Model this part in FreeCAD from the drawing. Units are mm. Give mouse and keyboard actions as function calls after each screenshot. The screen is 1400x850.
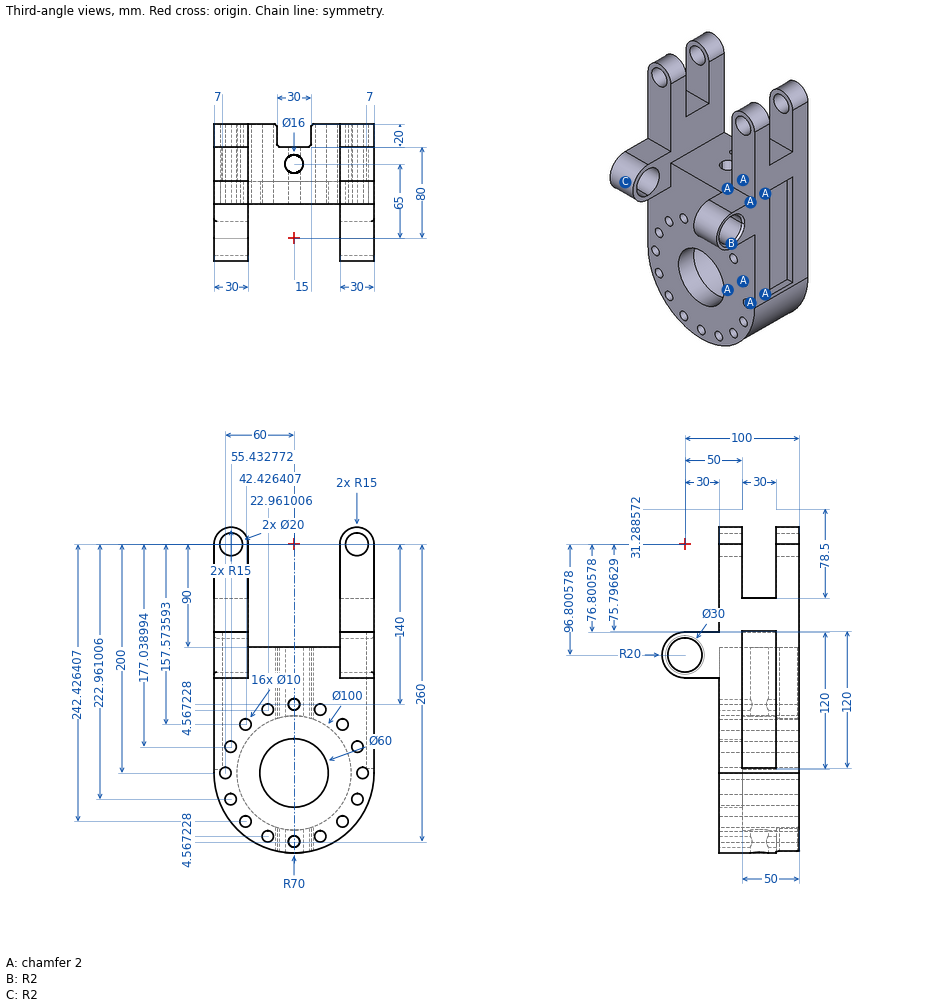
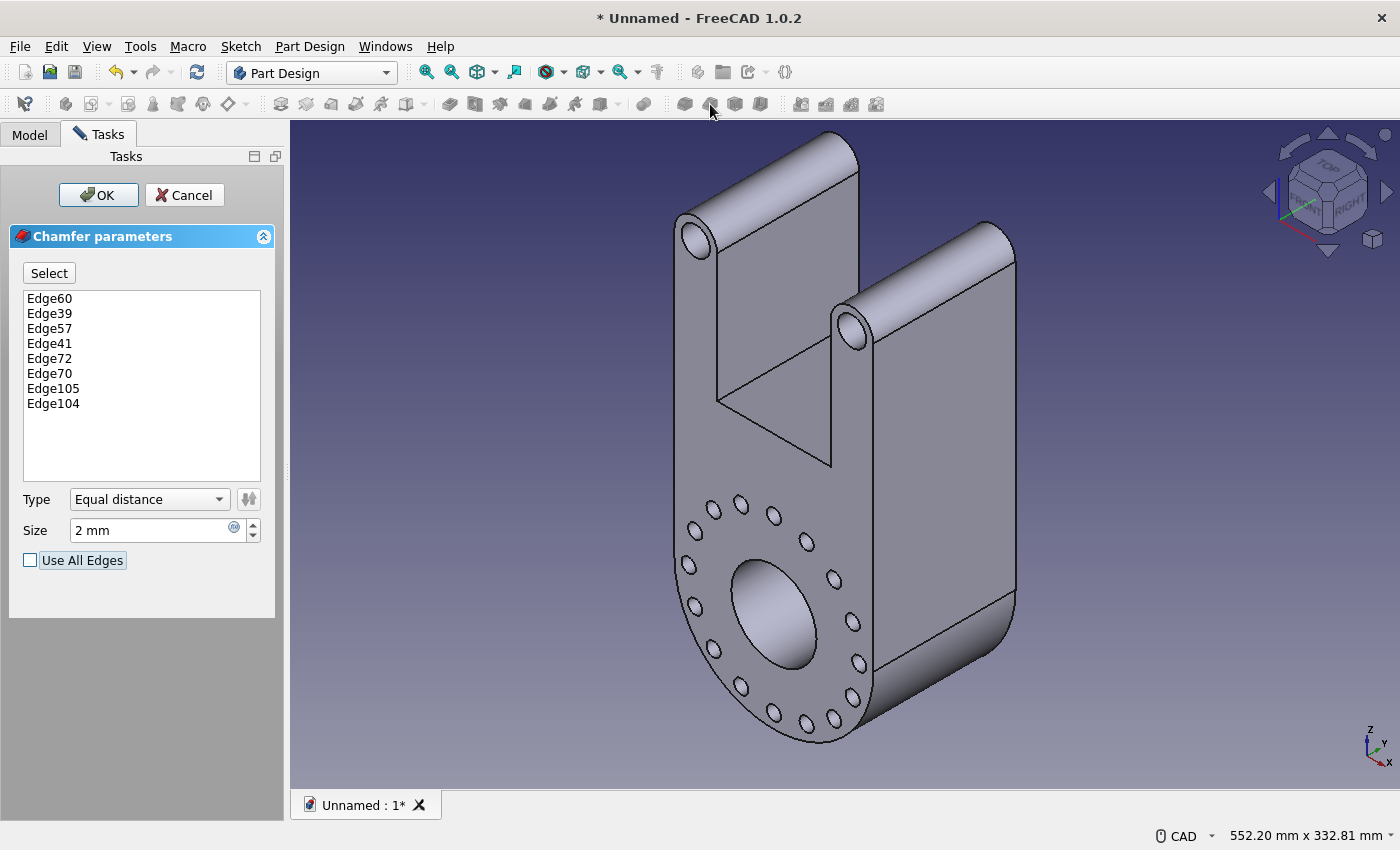
click(99, 195)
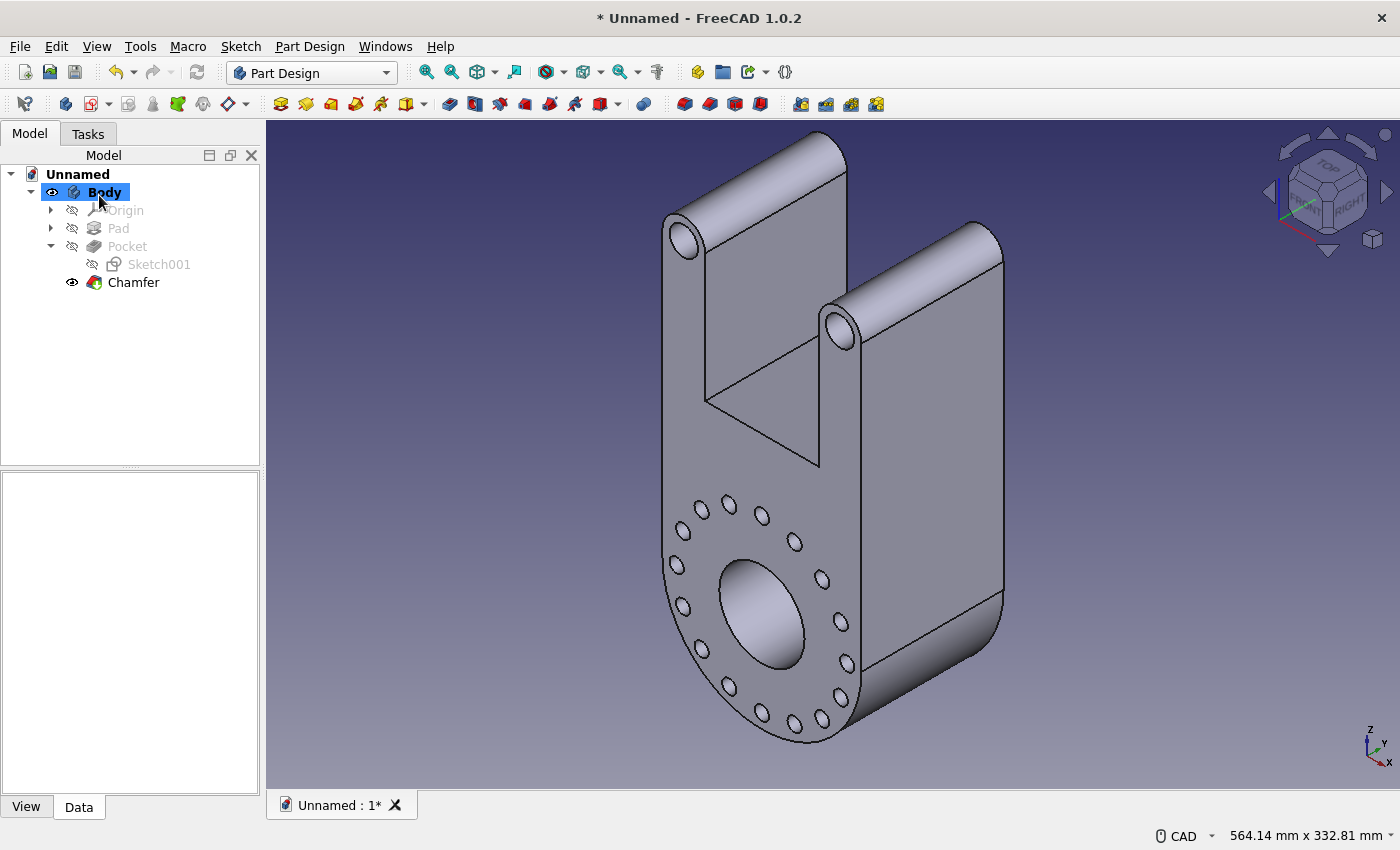
click(90, 104)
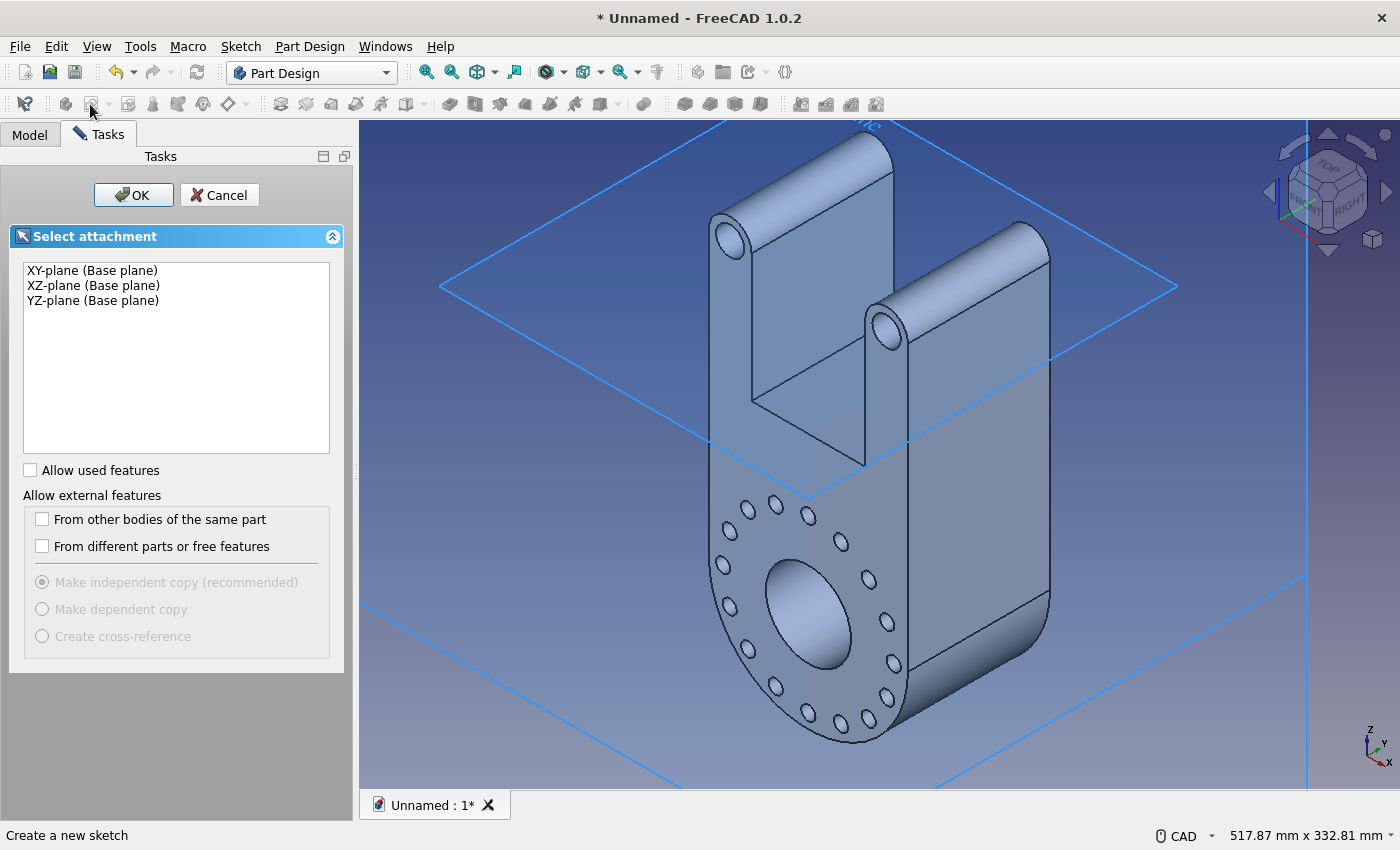
click(84, 286)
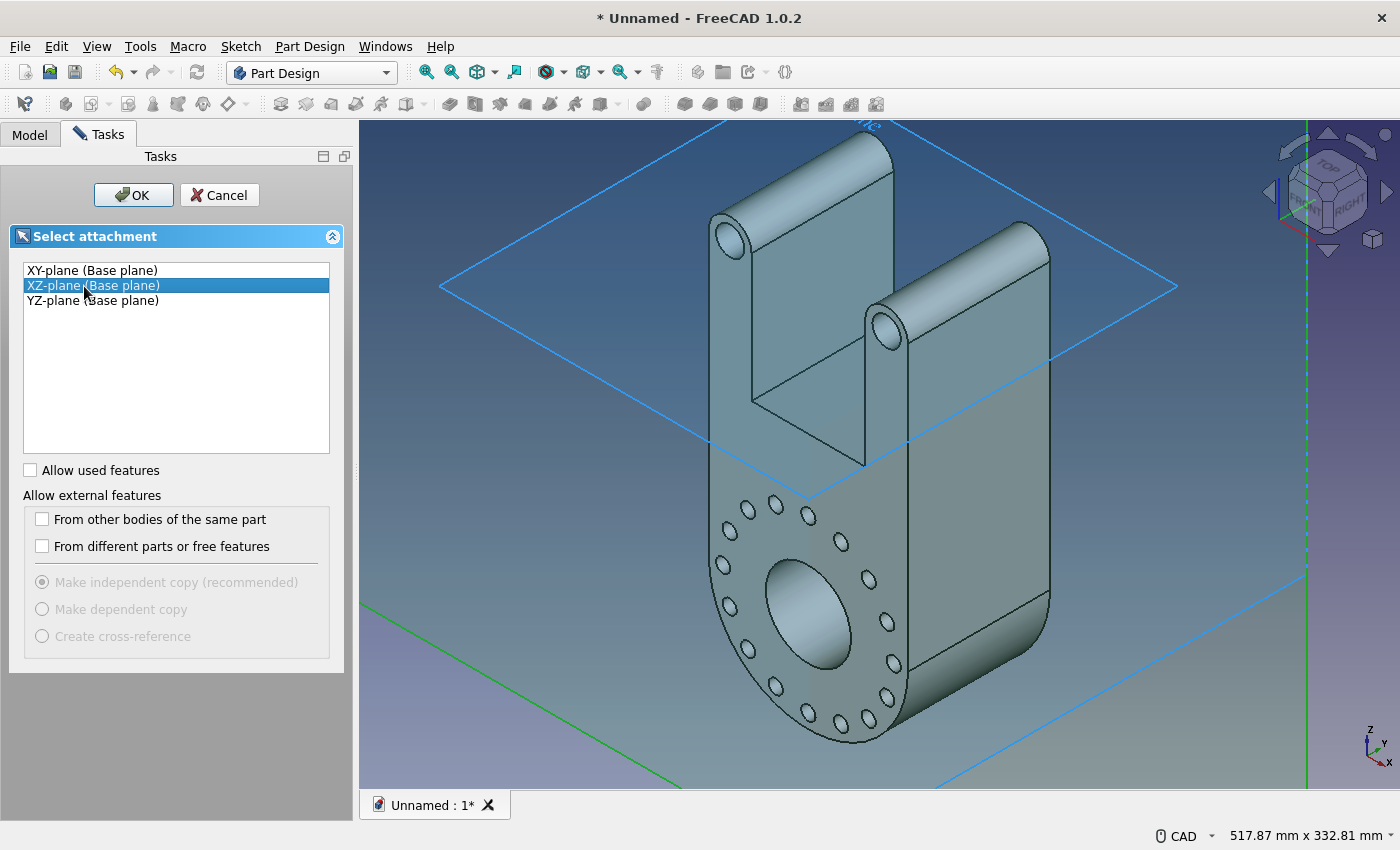
click(134, 195)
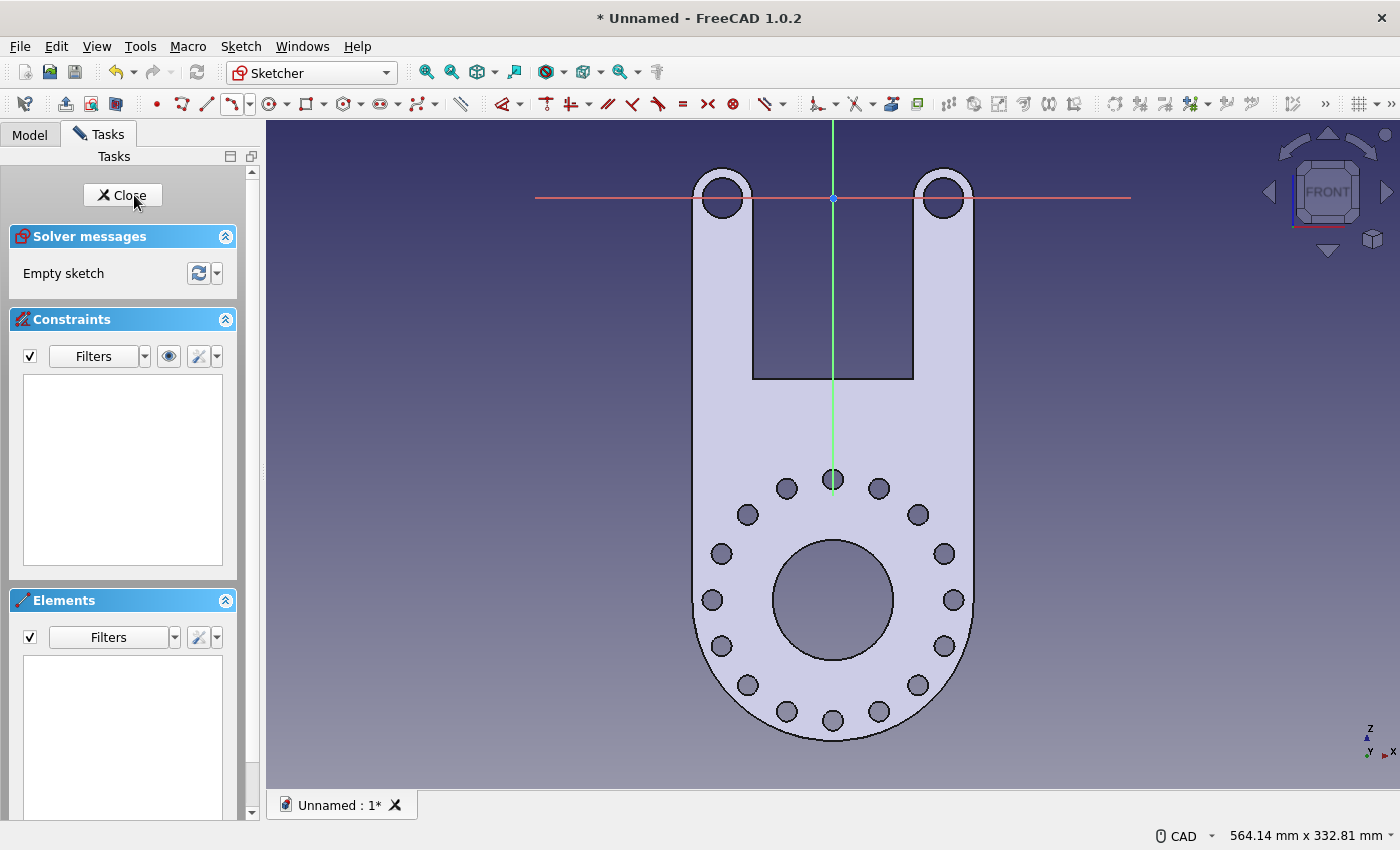
scroll(455, 455, down, 1)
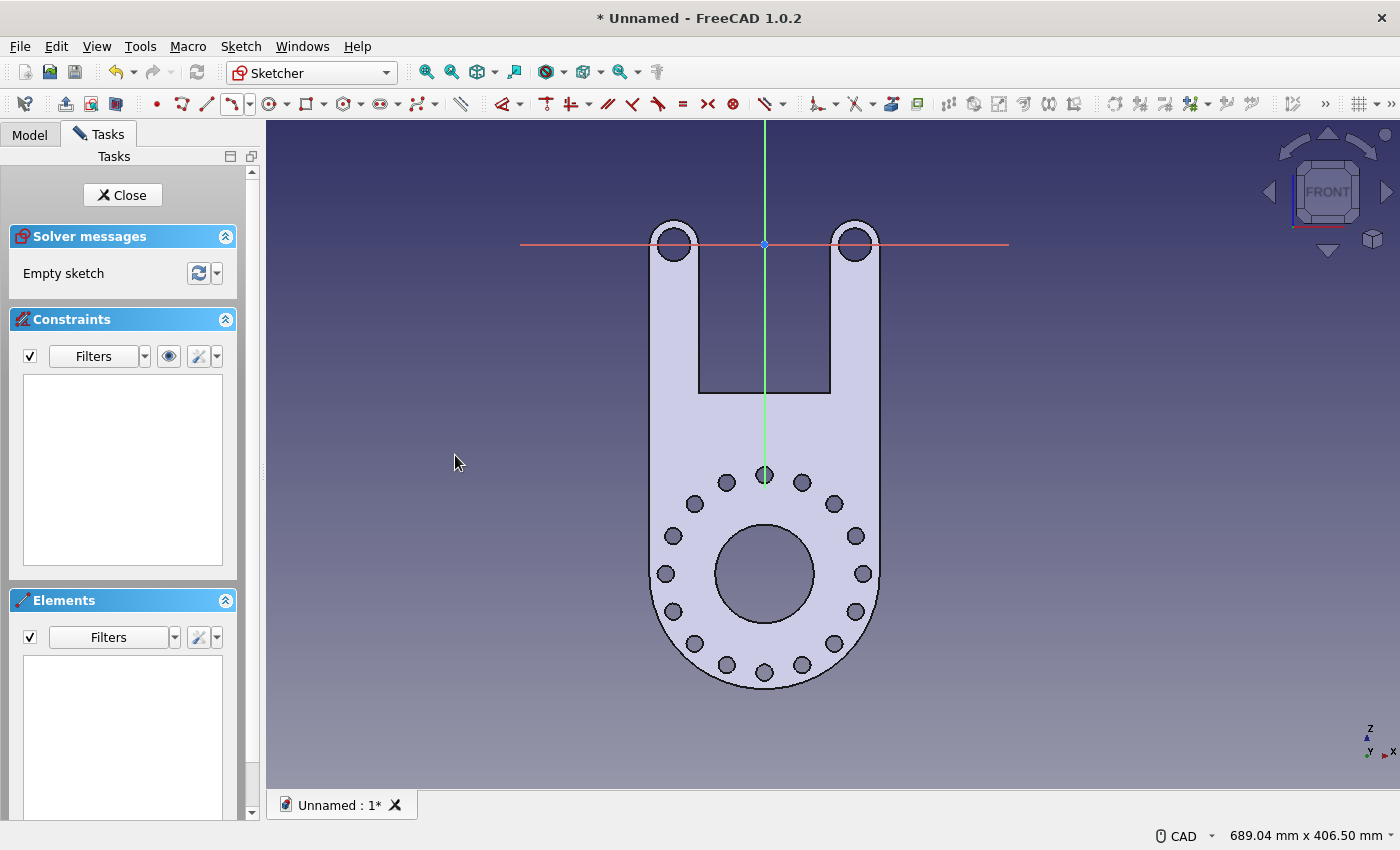
key(g)
key(l)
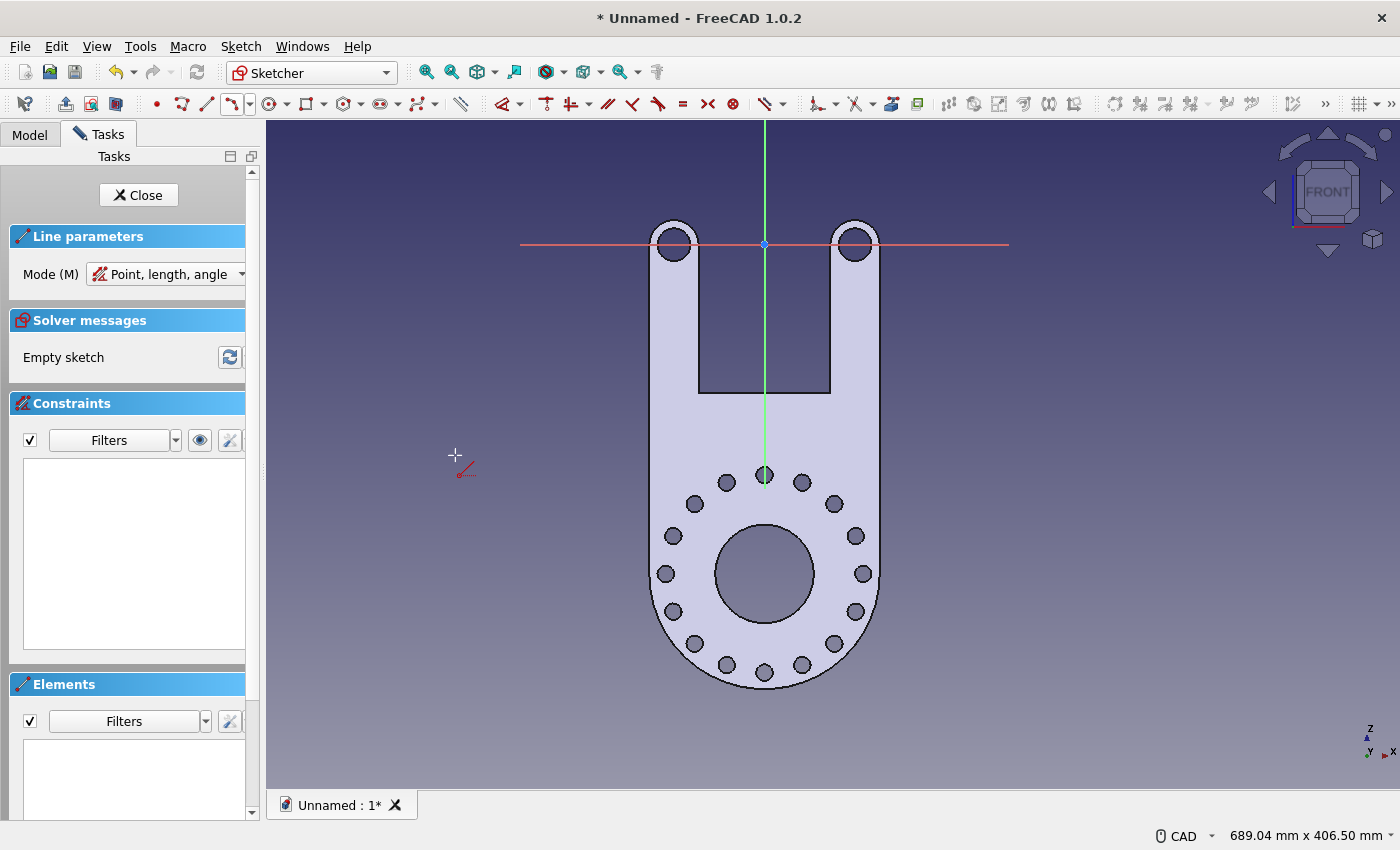
click(649, 245)
click(649, 574)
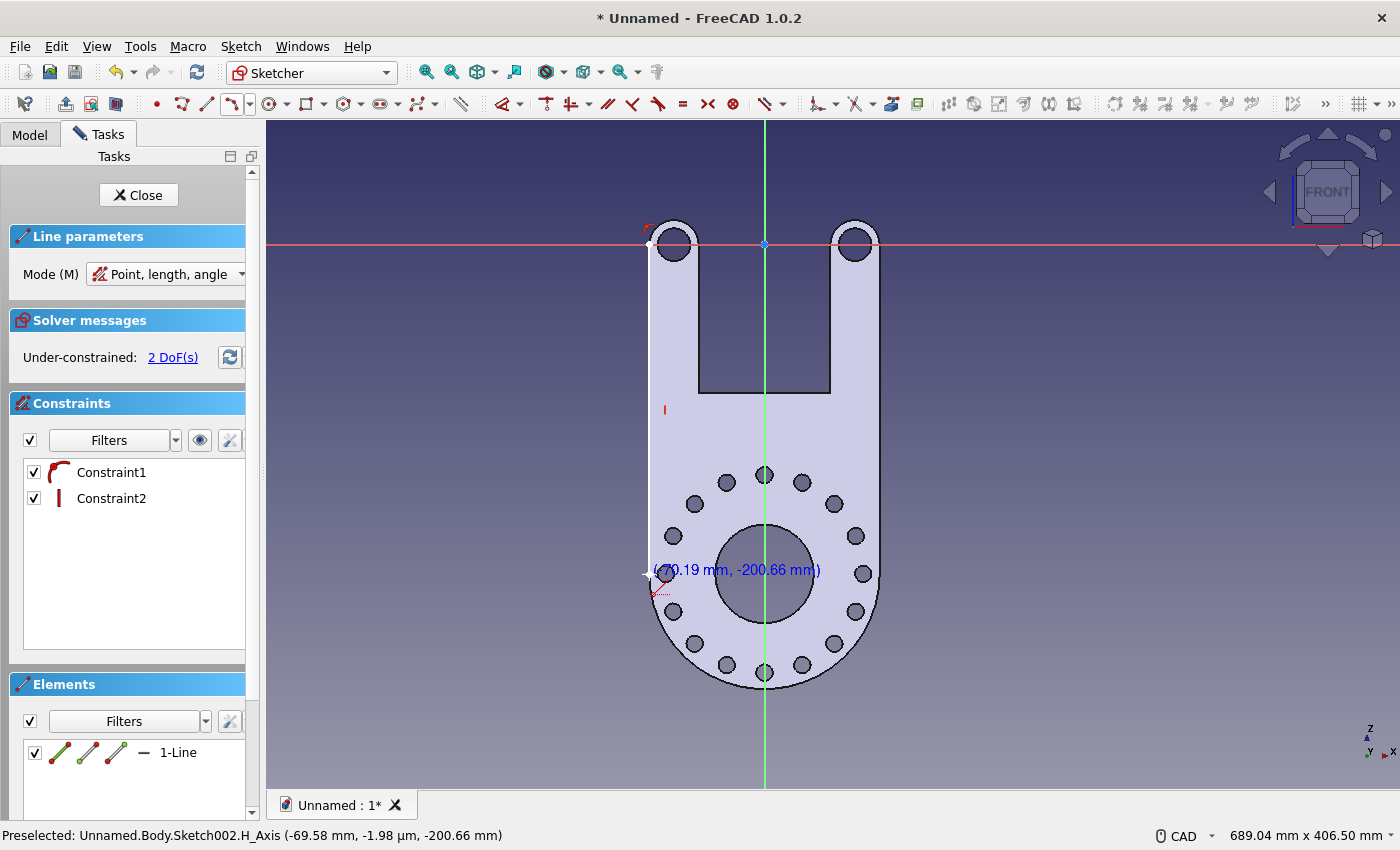
click(880, 574)
click(880, 245)